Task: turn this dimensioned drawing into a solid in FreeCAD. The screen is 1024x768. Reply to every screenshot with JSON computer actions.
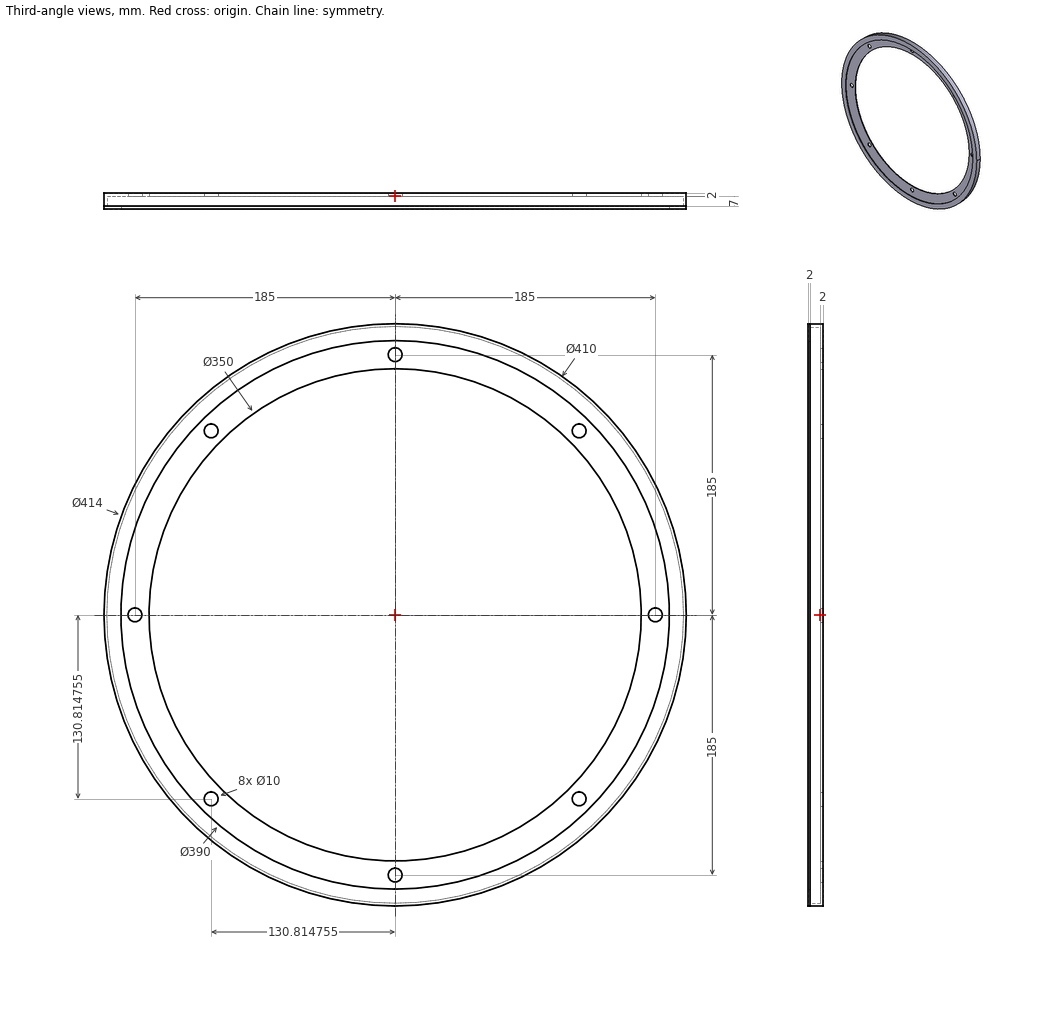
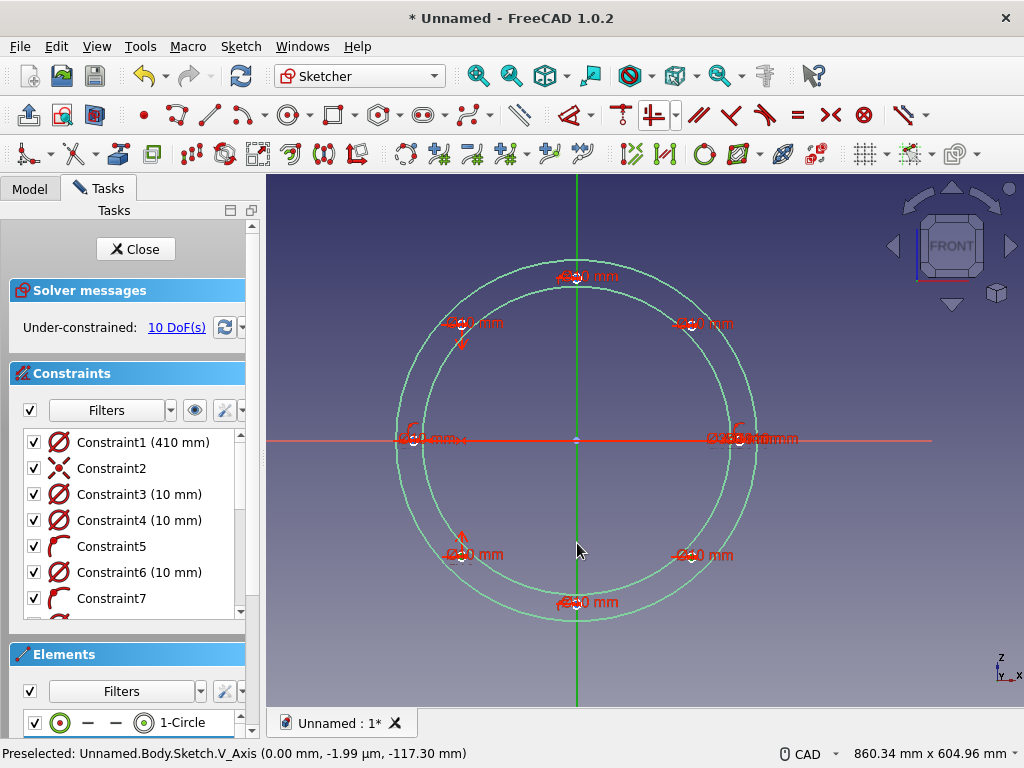
{"action": "left_click", "coordinate": [831, 116]}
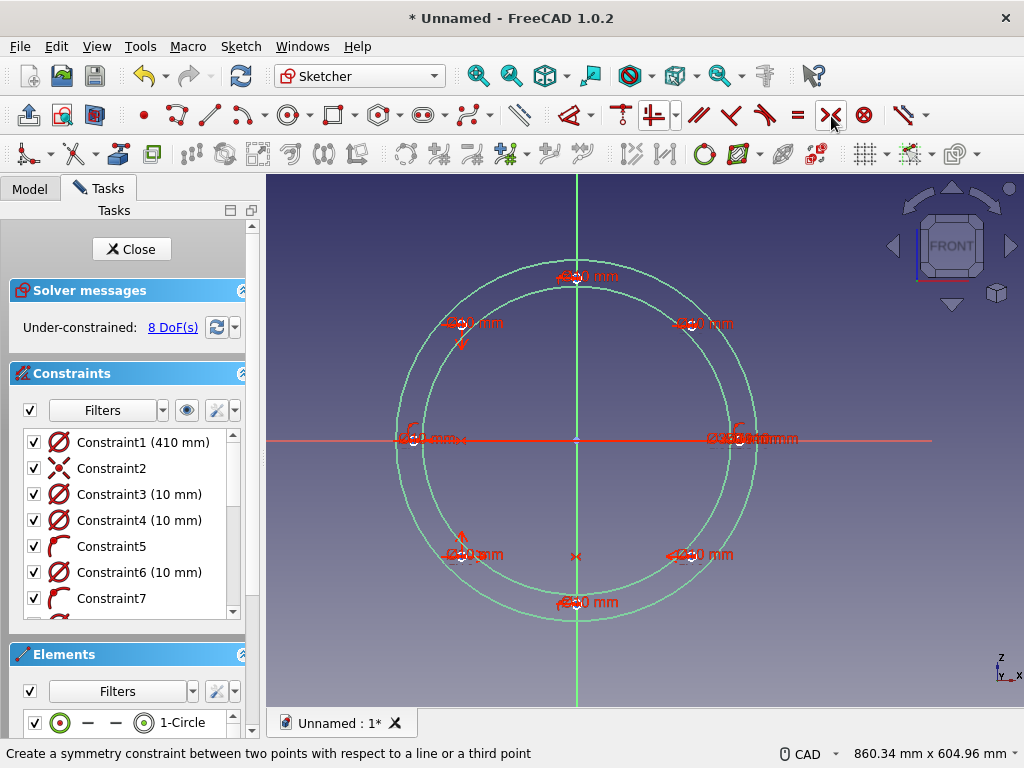
{"action": "left_click", "coordinate": [462, 325]}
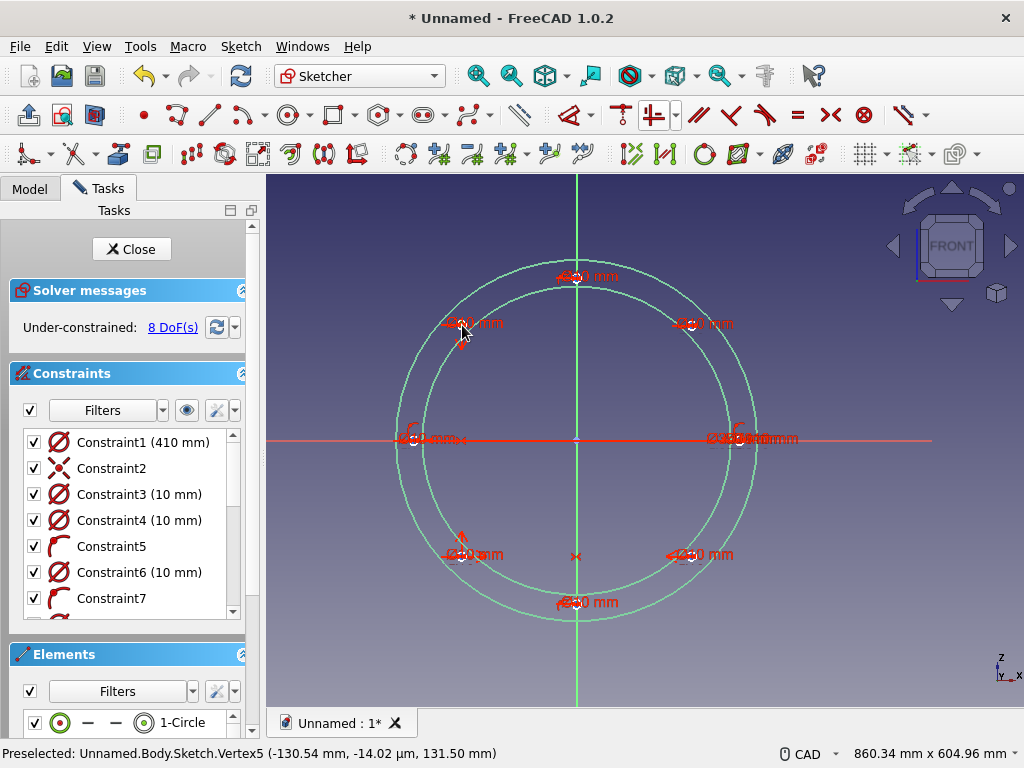
{"action": "left_click", "coordinate": [692, 326]}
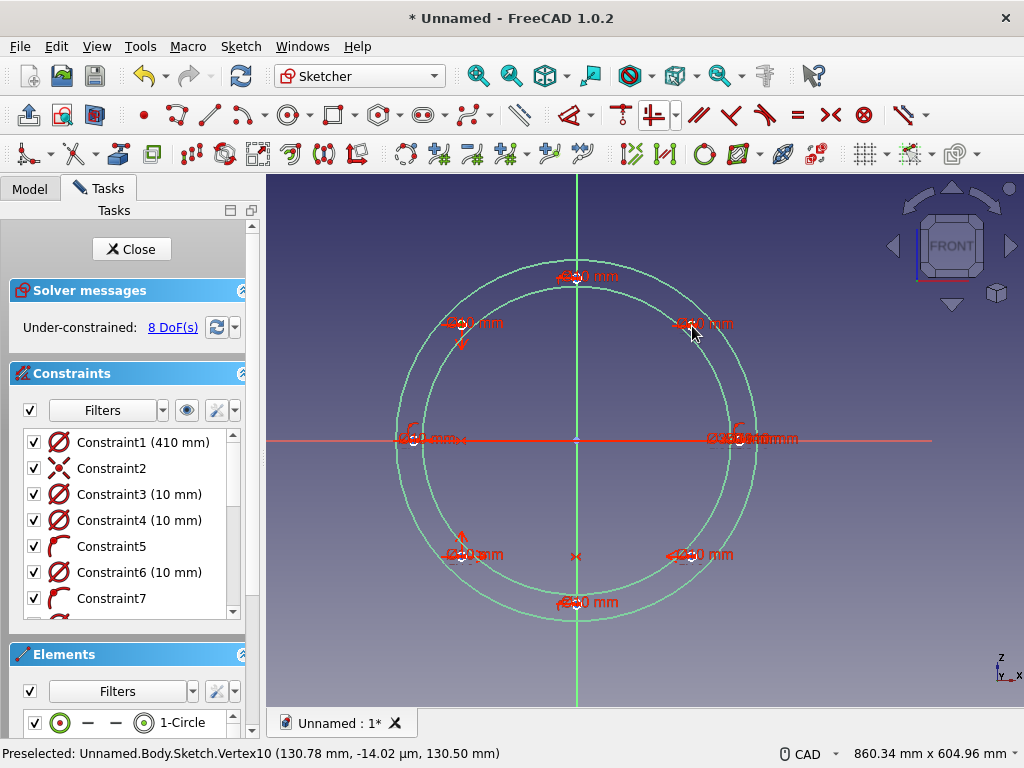
{"action": "left_click", "coordinate": [577, 543]}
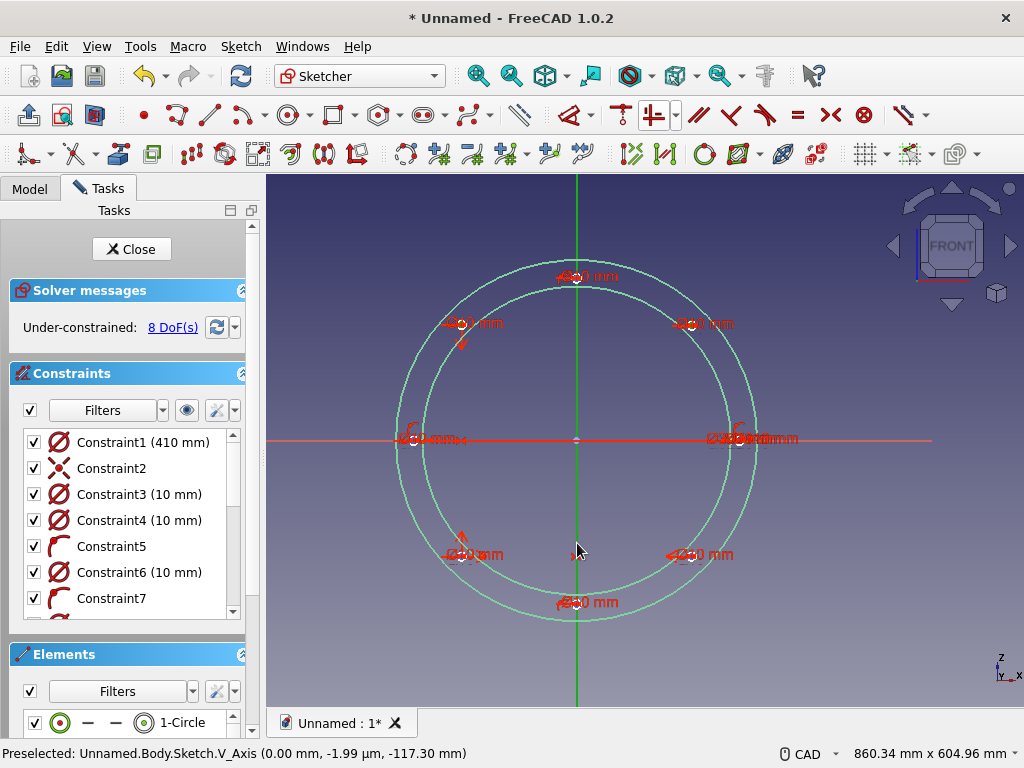
{"action": "left_click", "coordinate": [831, 116]}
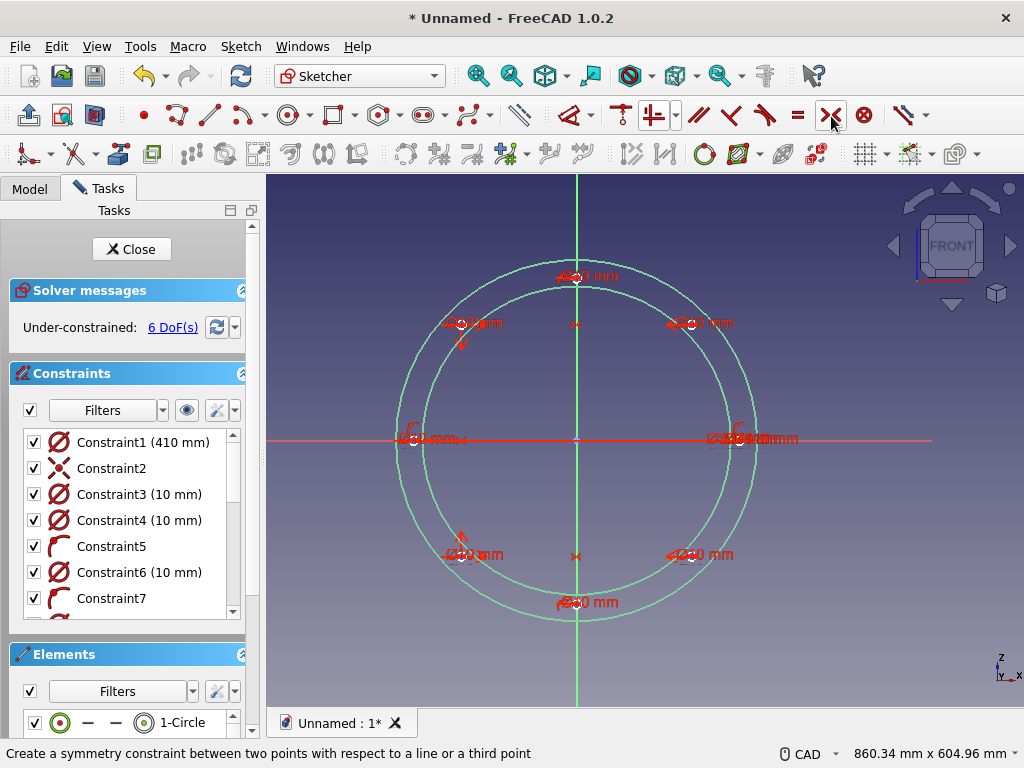
{"action": "left_click", "coordinate": [577, 604]}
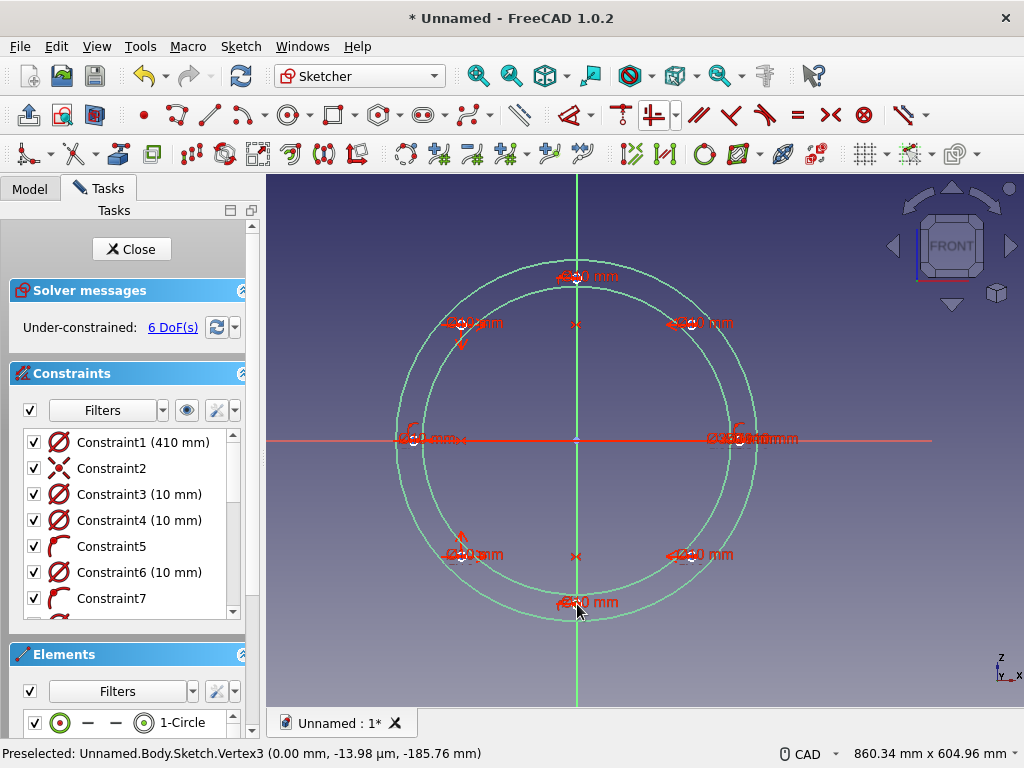
{"action": "key", "text": "i"}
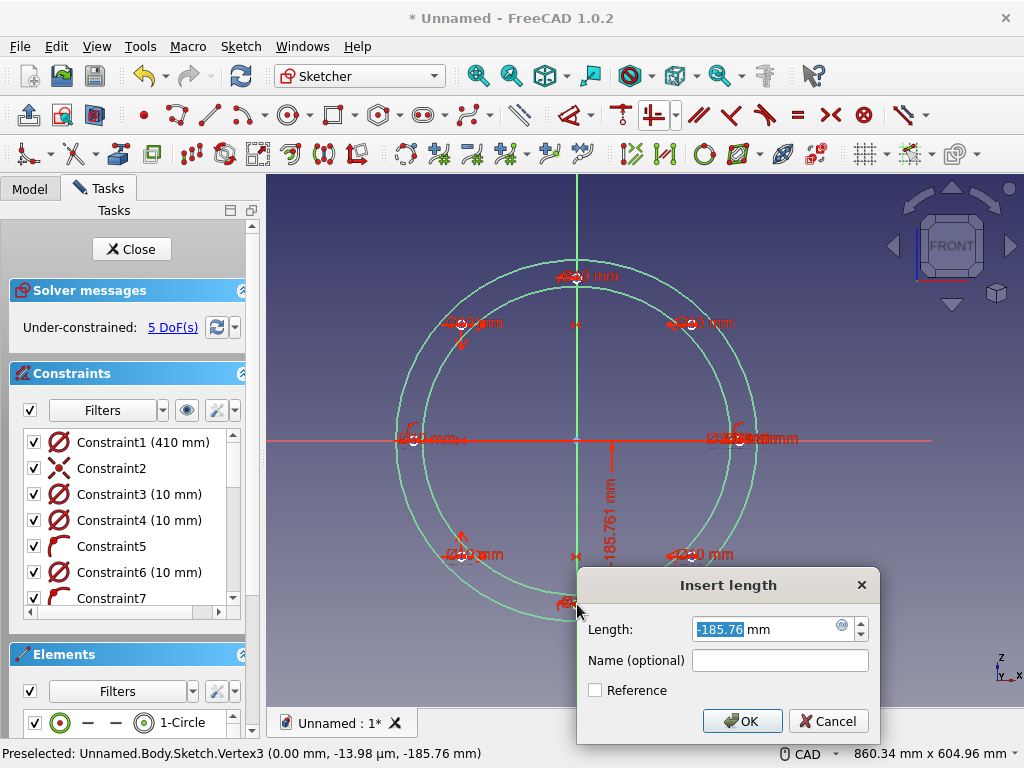
{"action": "type", "text": "-185"}
{"action": "key", "text": "Return"}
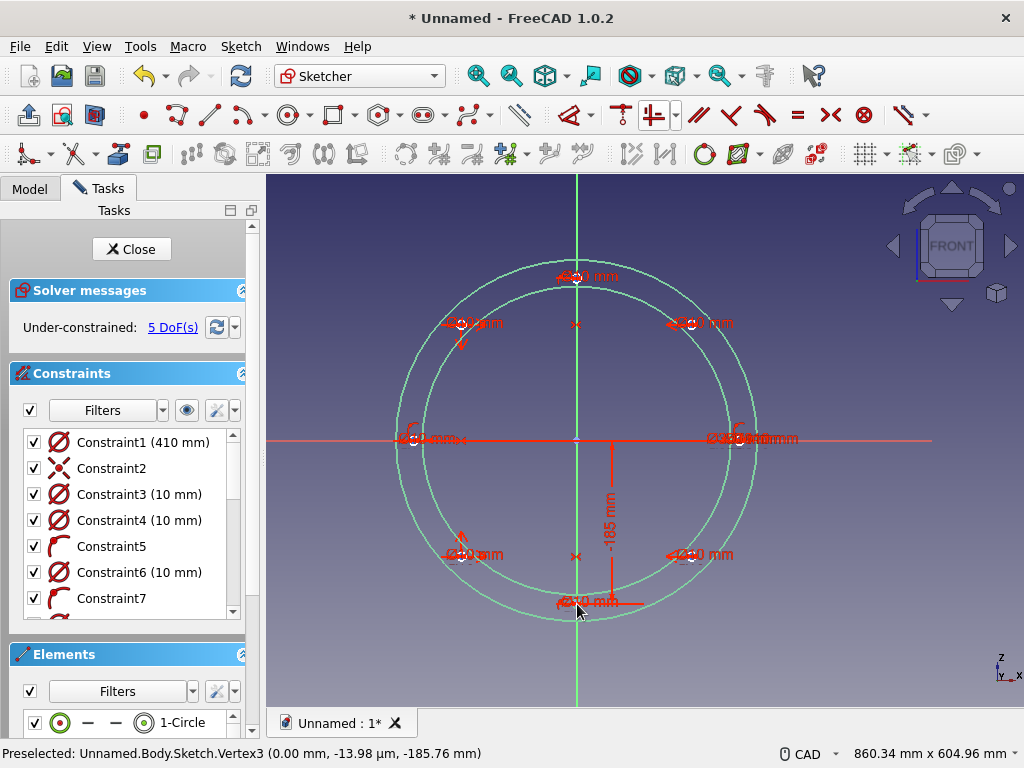
{"action": "left_click", "coordinate": [414, 441]}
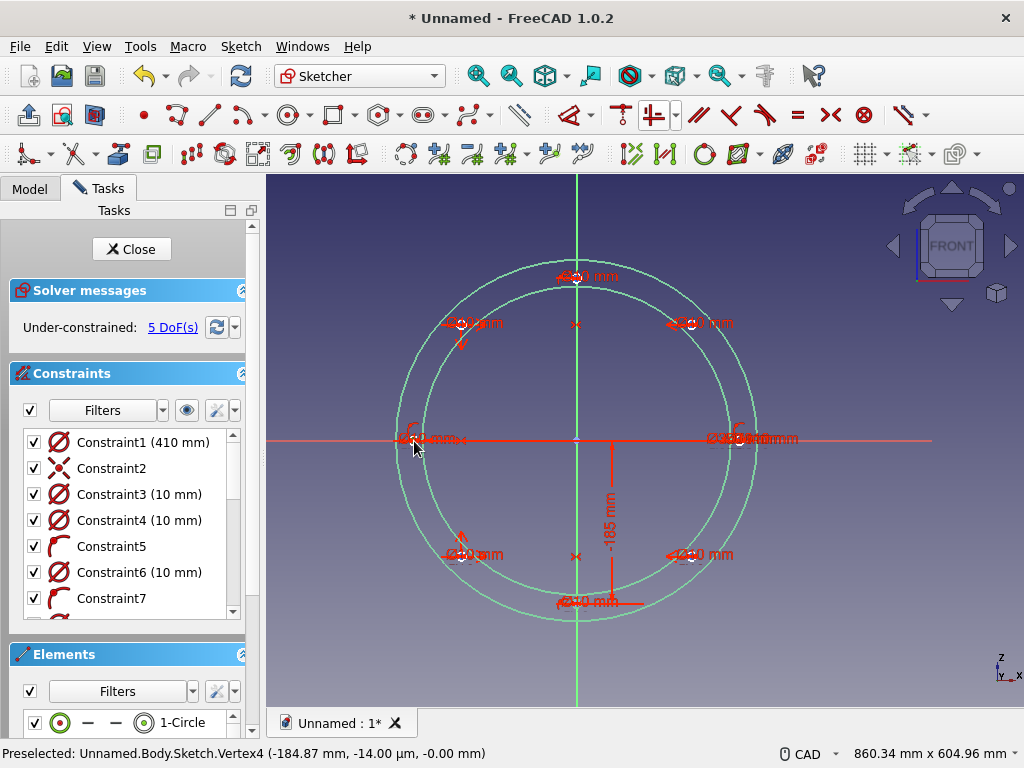
{"action": "left_click", "coordinate": [590, 116]}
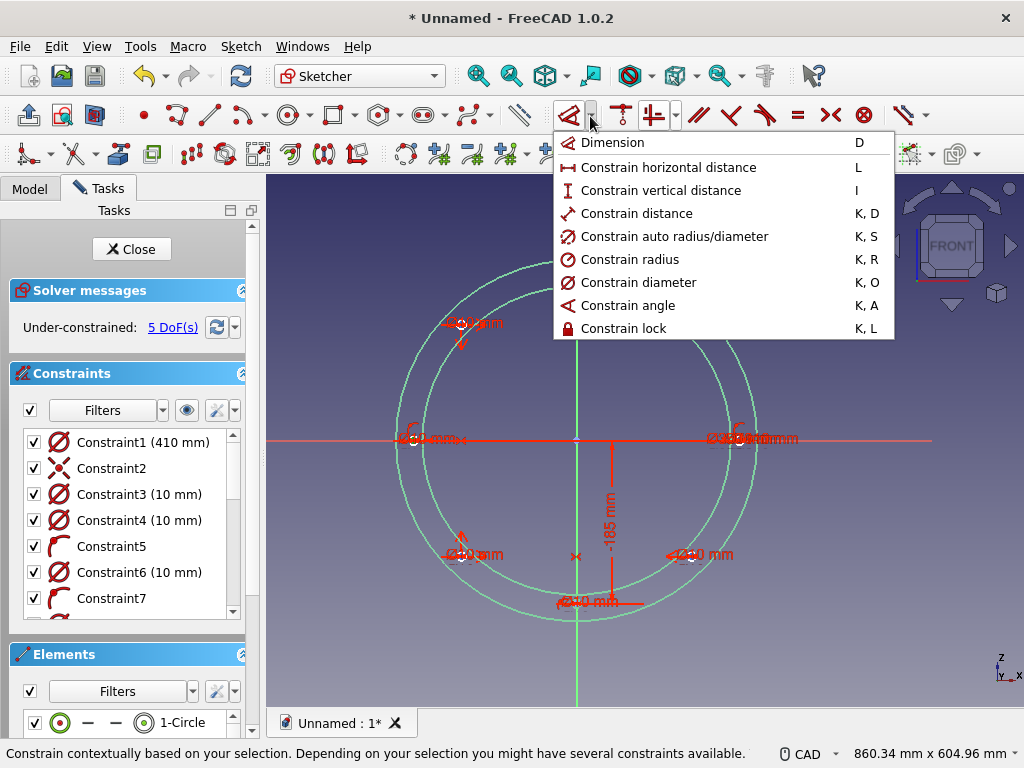
{"action": "left_click", "coordinate": [724, 168]}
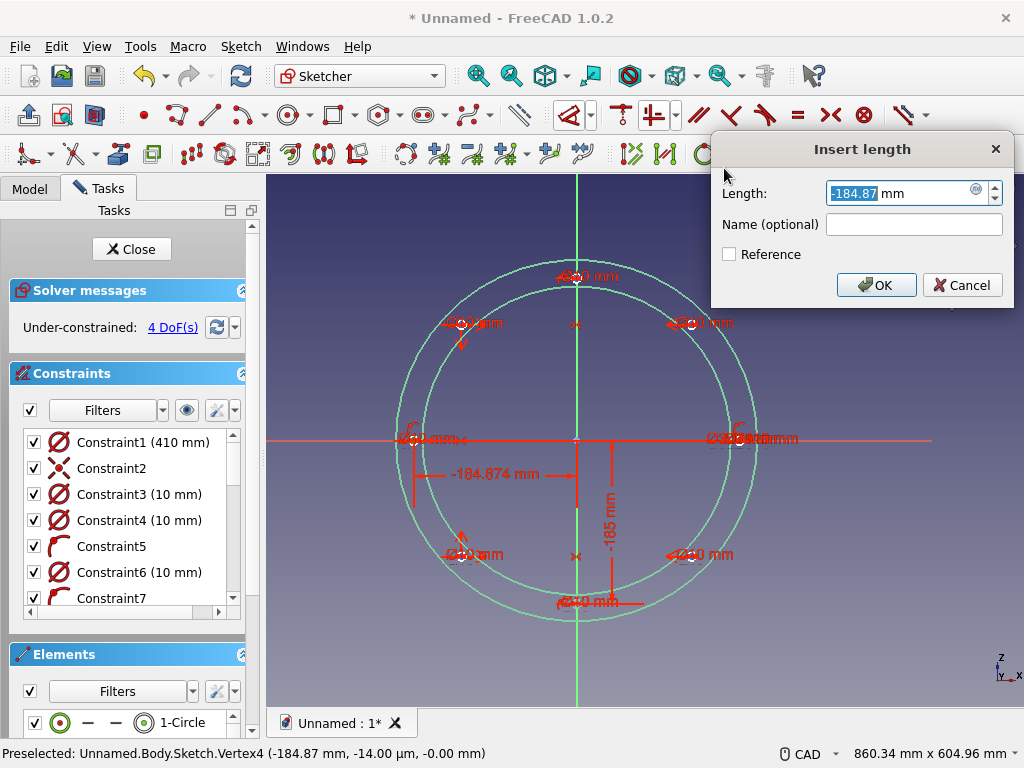
{"action": "type", "text": "-185"}
{"action": "key", "text": "Return"}